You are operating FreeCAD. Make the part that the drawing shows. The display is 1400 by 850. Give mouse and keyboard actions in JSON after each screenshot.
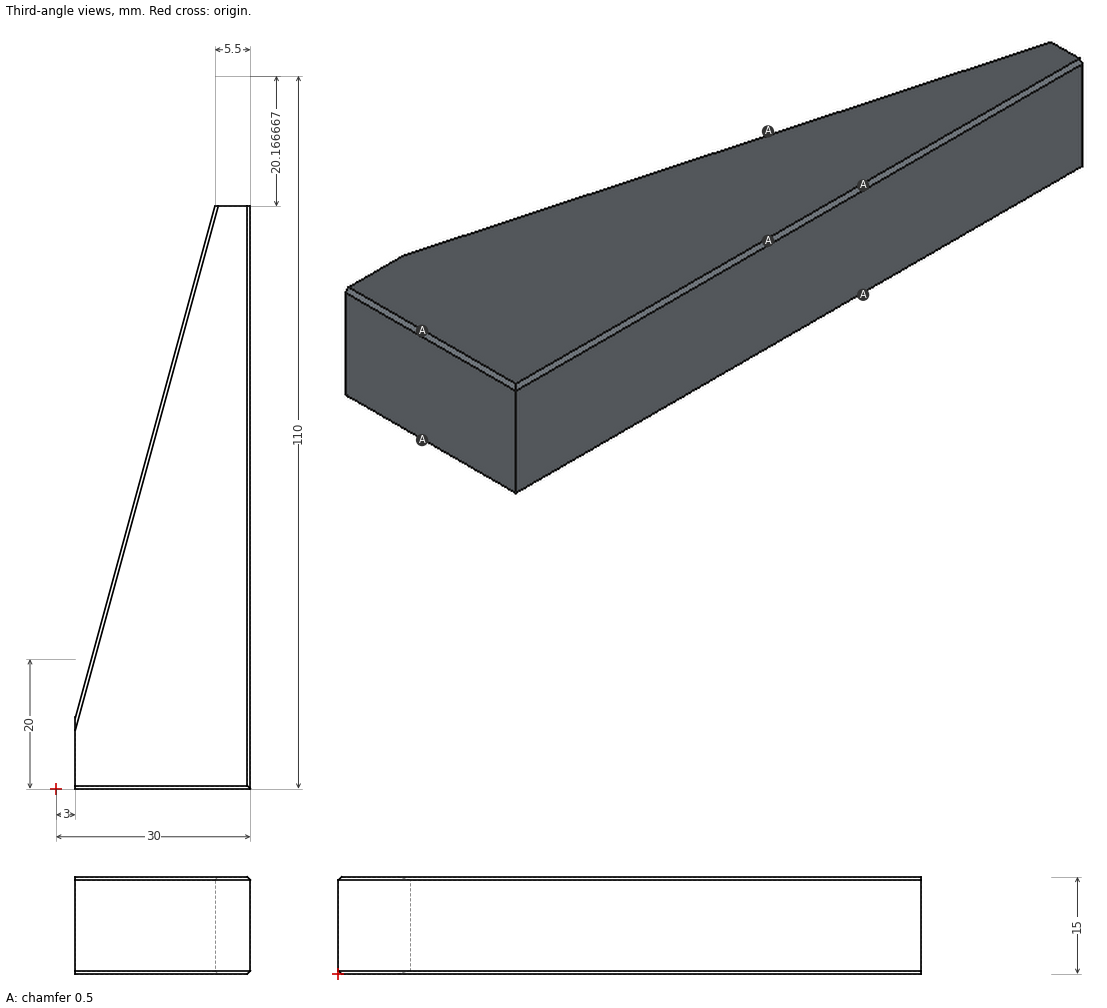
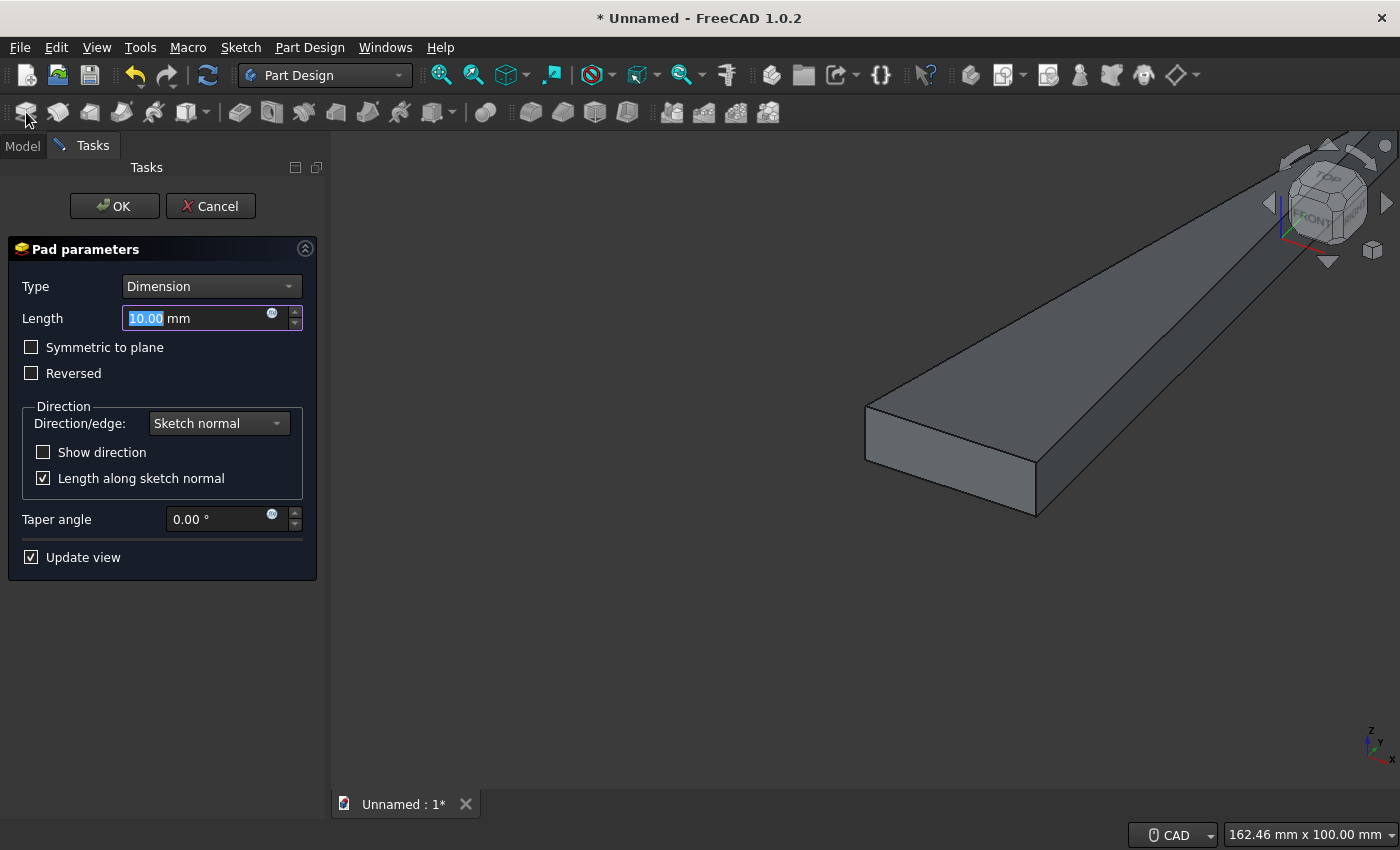
{"action": "type", "text": "15"}
{"action": "key", "text": "Tab"}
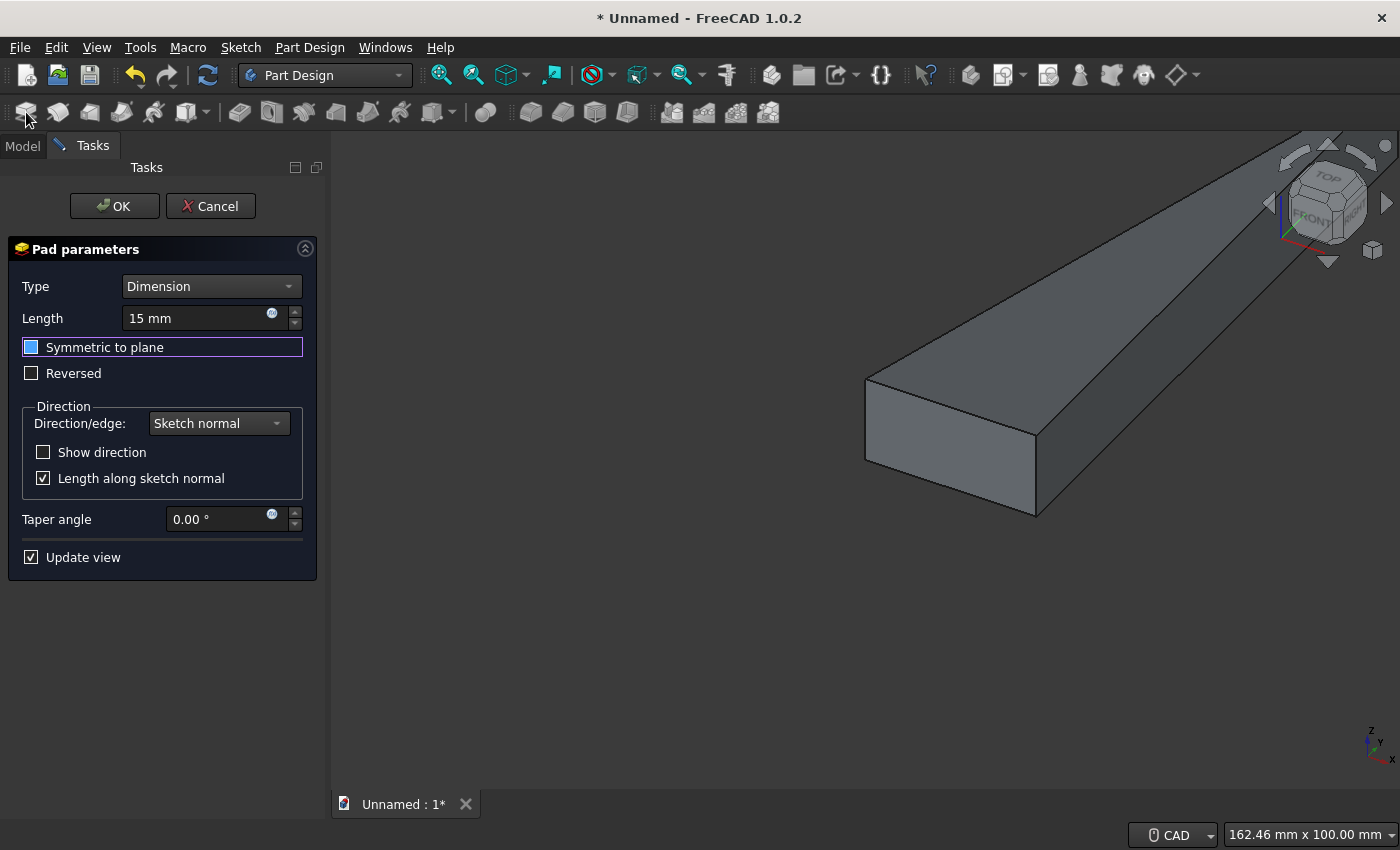
{"action": "left_click", "coordinate": [115, 206]}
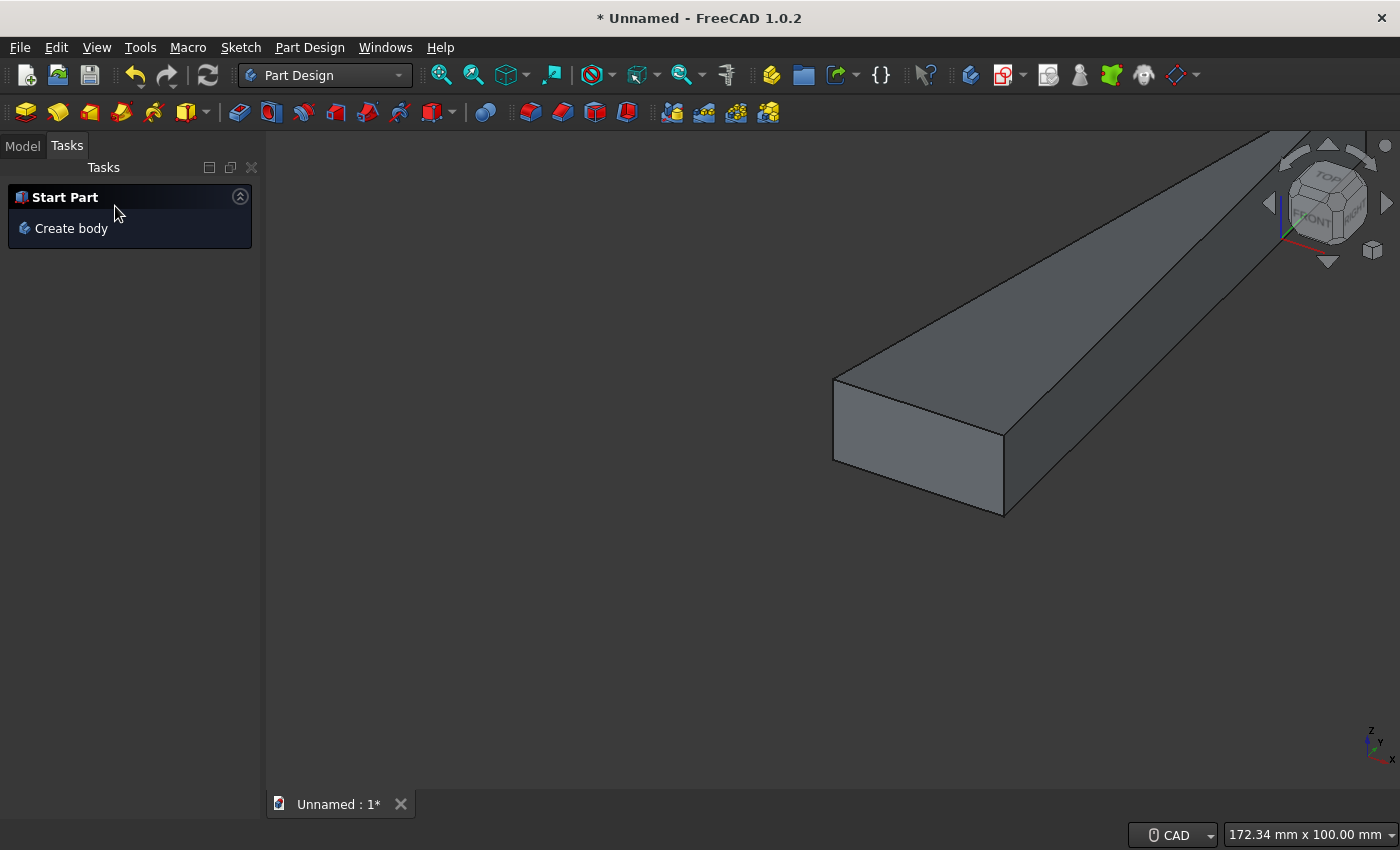
{"action": "left_click", "coordinate": [442, 76]}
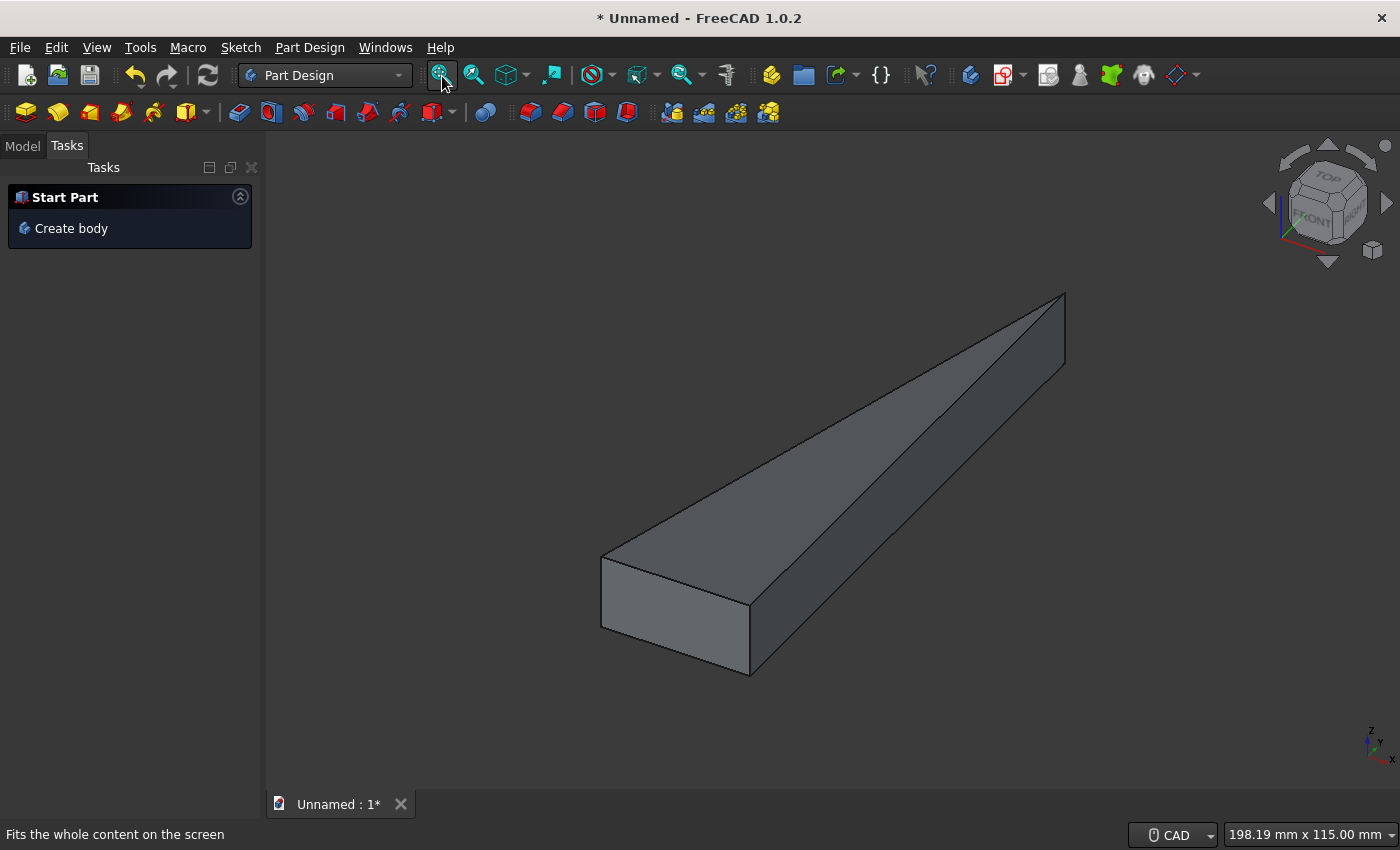
{"action": "left_click", "coordinate": [764, 520]}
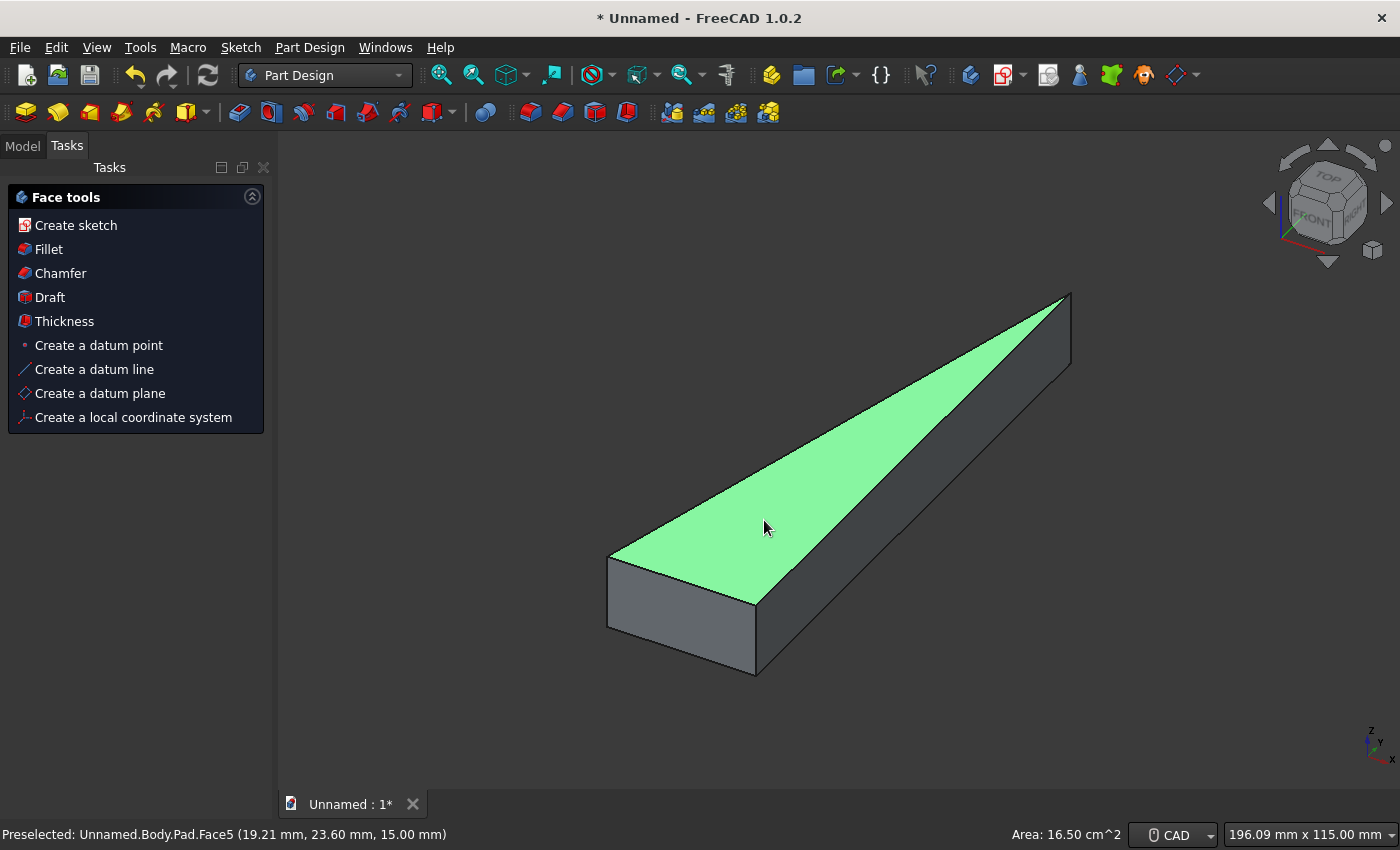
{"action": "key", "text": "0"}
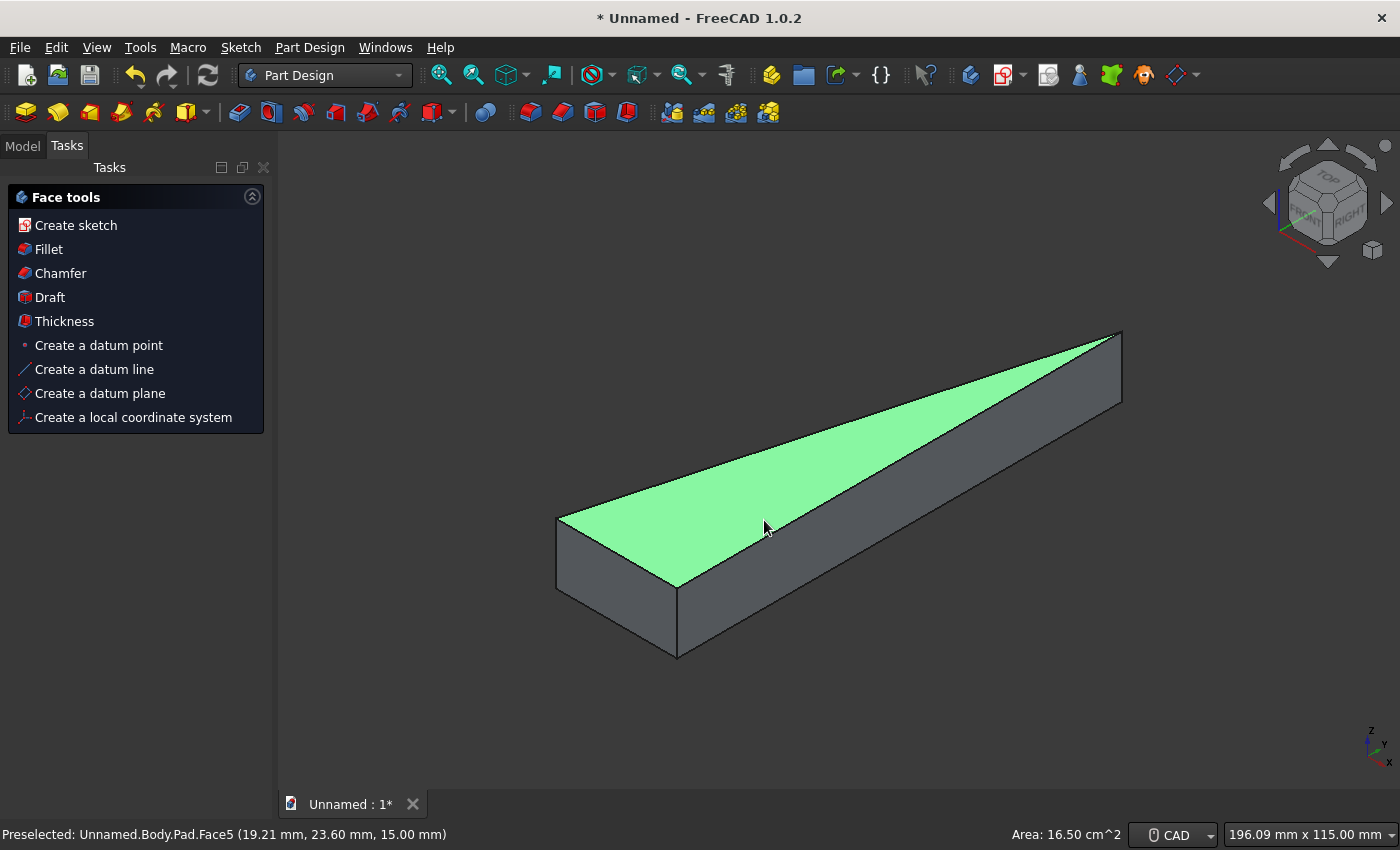
{"action": "key", "text": "2"}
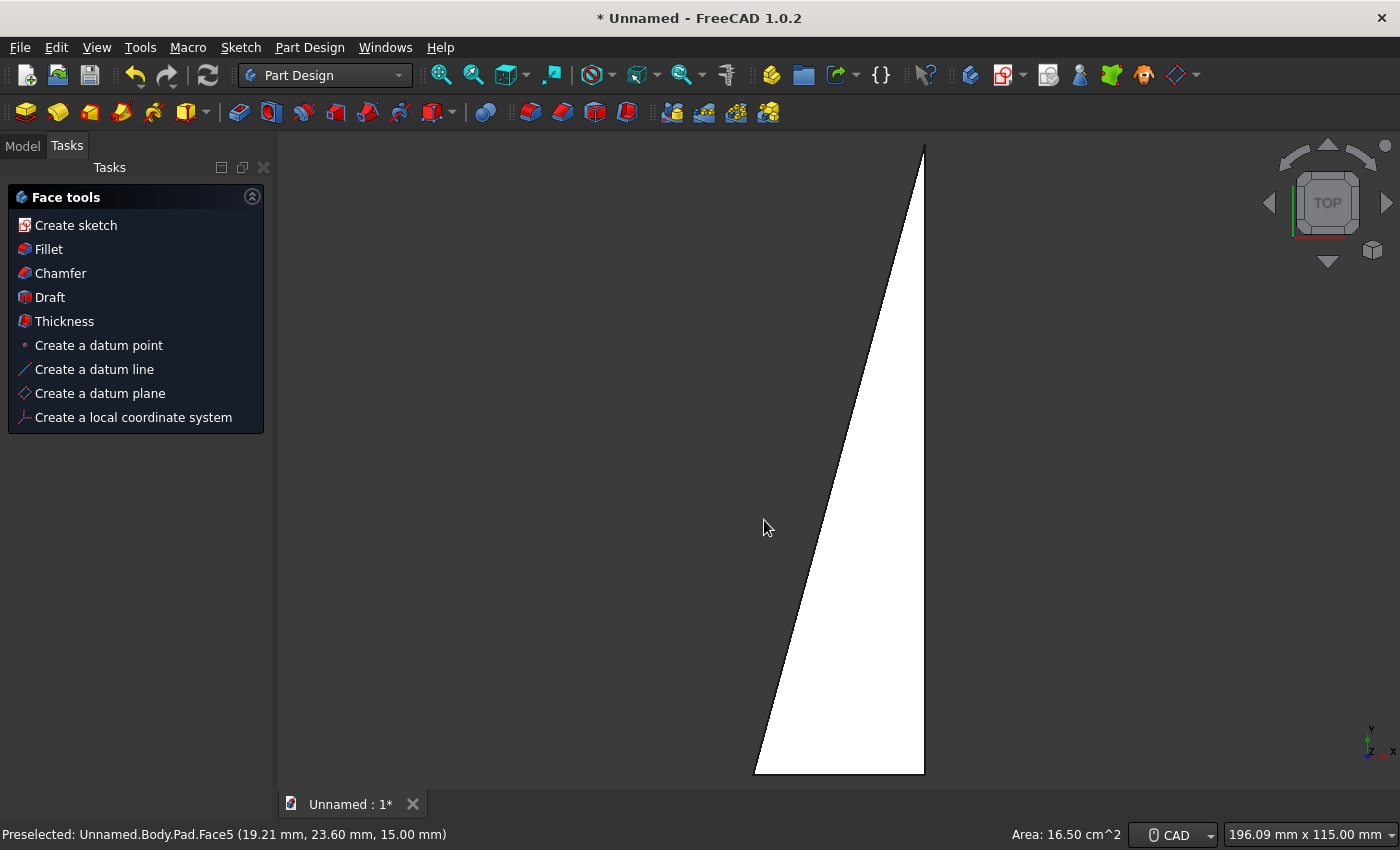
{"action": "key", "text": "1"}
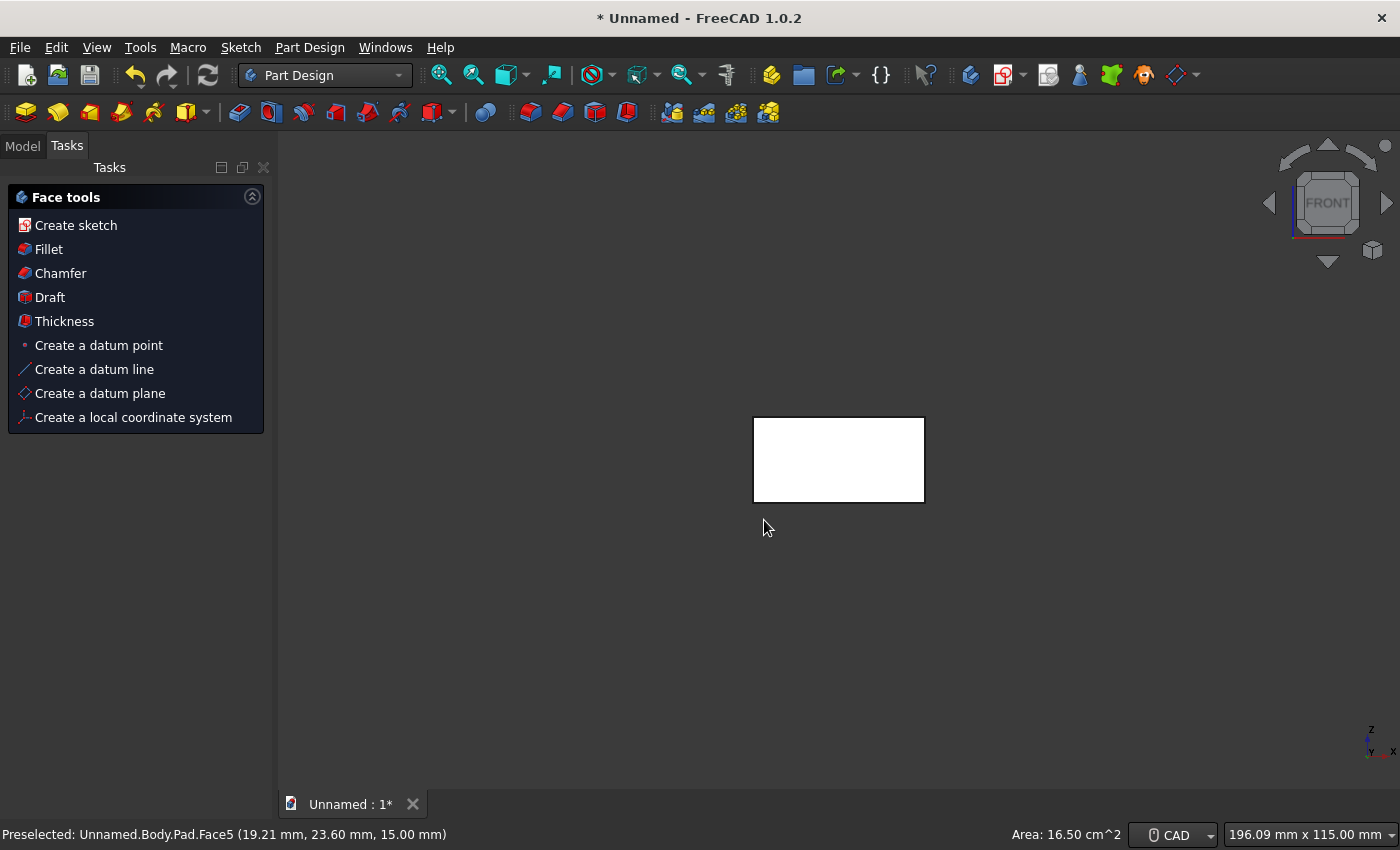
{"action": "left_click", "coordinate": [442, 76]}